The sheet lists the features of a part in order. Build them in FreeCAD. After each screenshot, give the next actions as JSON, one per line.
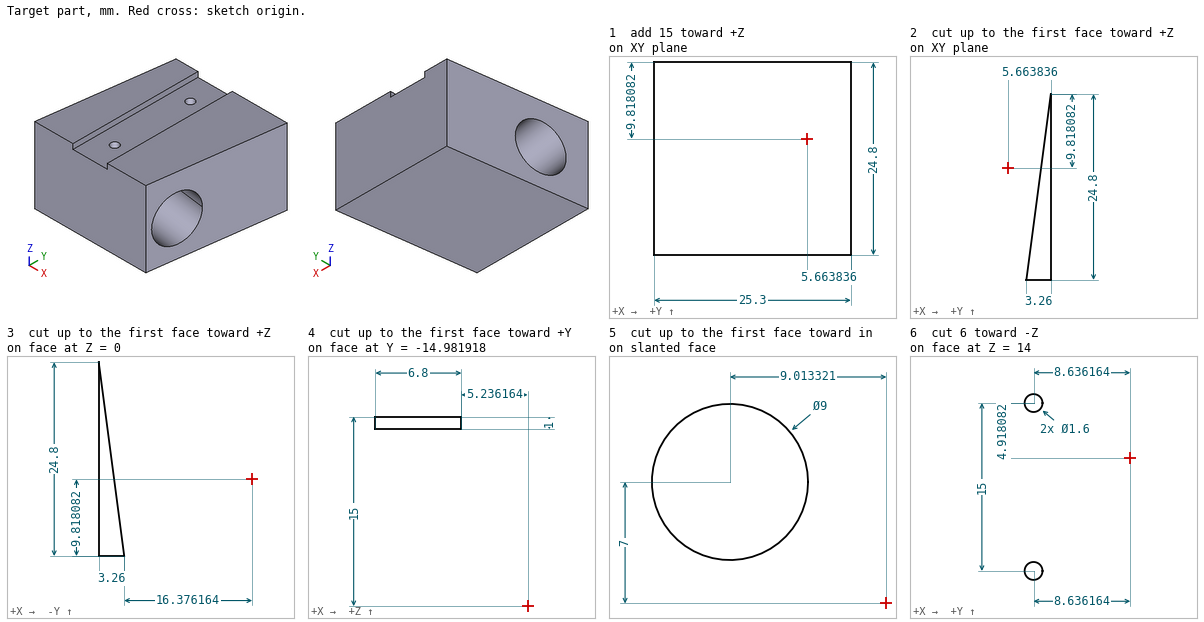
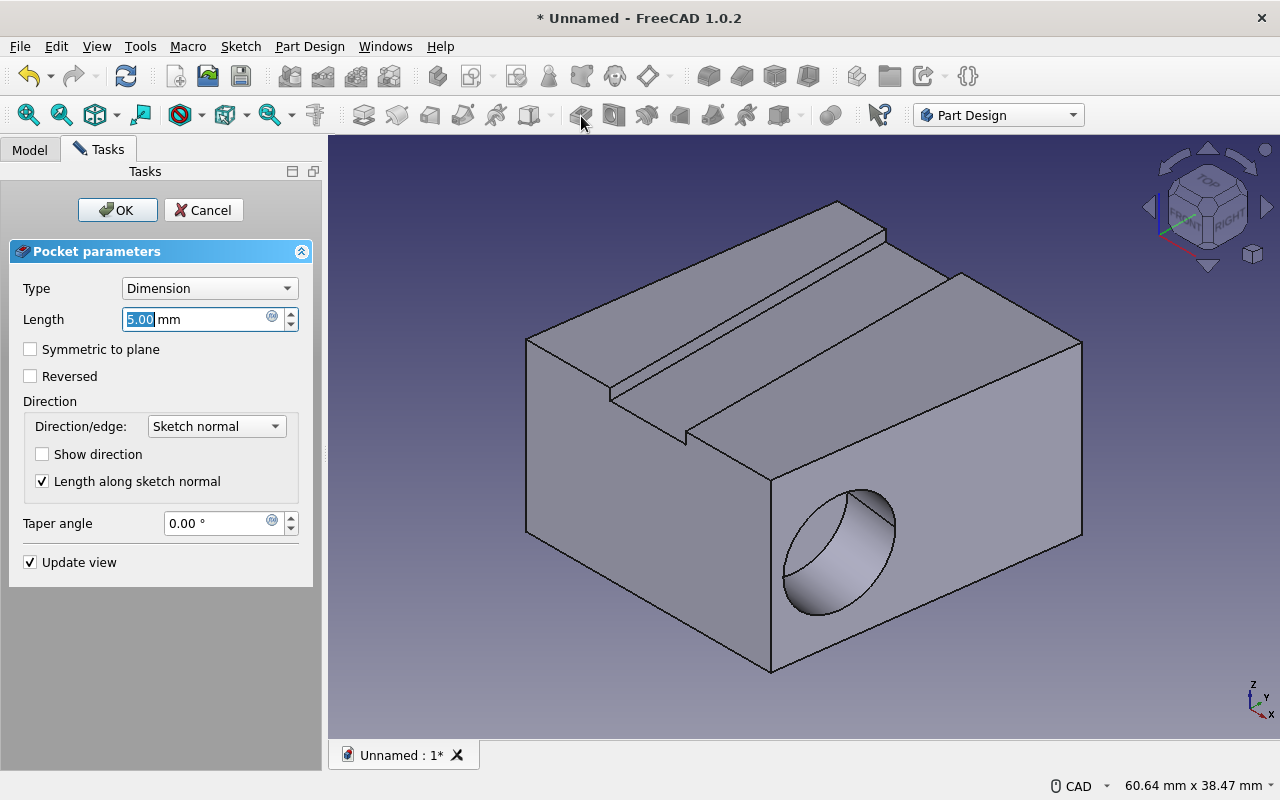
{"action": "left_click", "coordinate": [210, 288]}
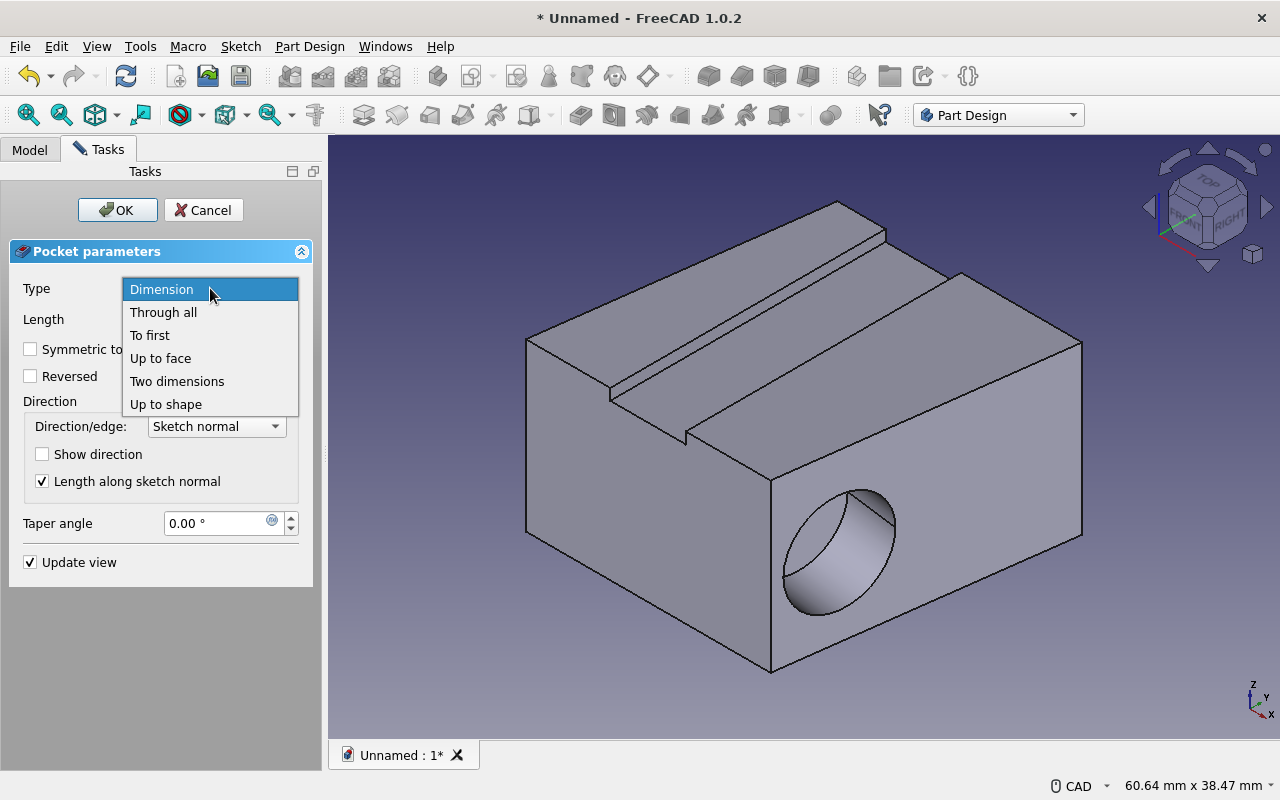
{"action": "left_click", "coordinate": [208, 336]}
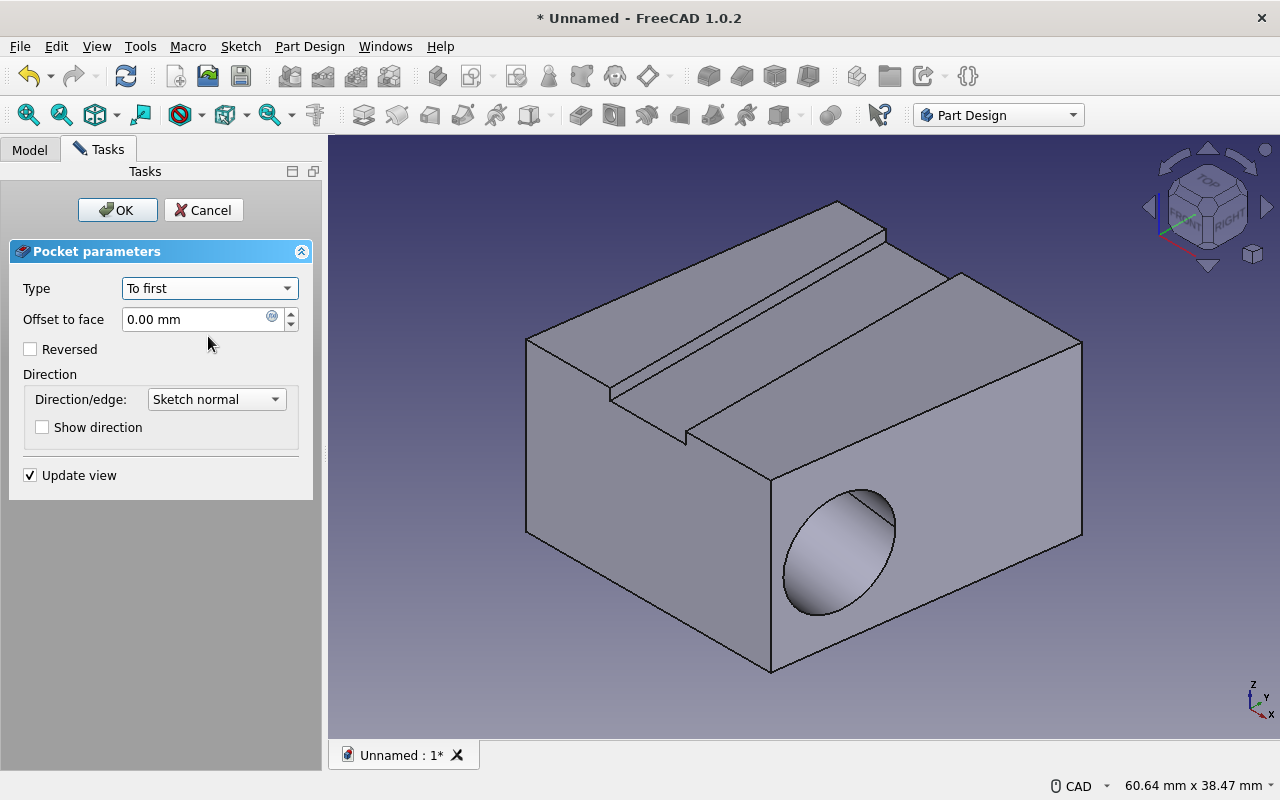
{"action": "left_click", "coordinate": [118, 210]}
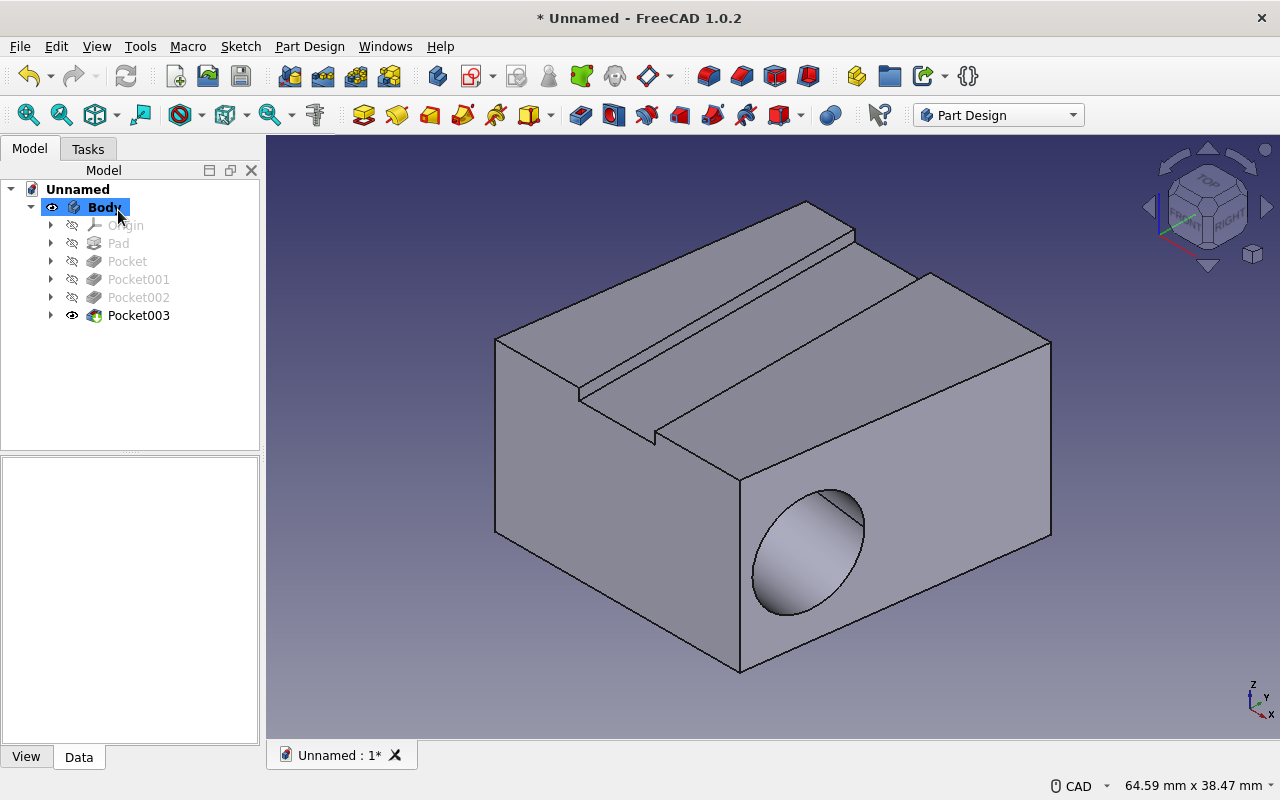
{"action": "left_click", "coordinate": [833, 297]}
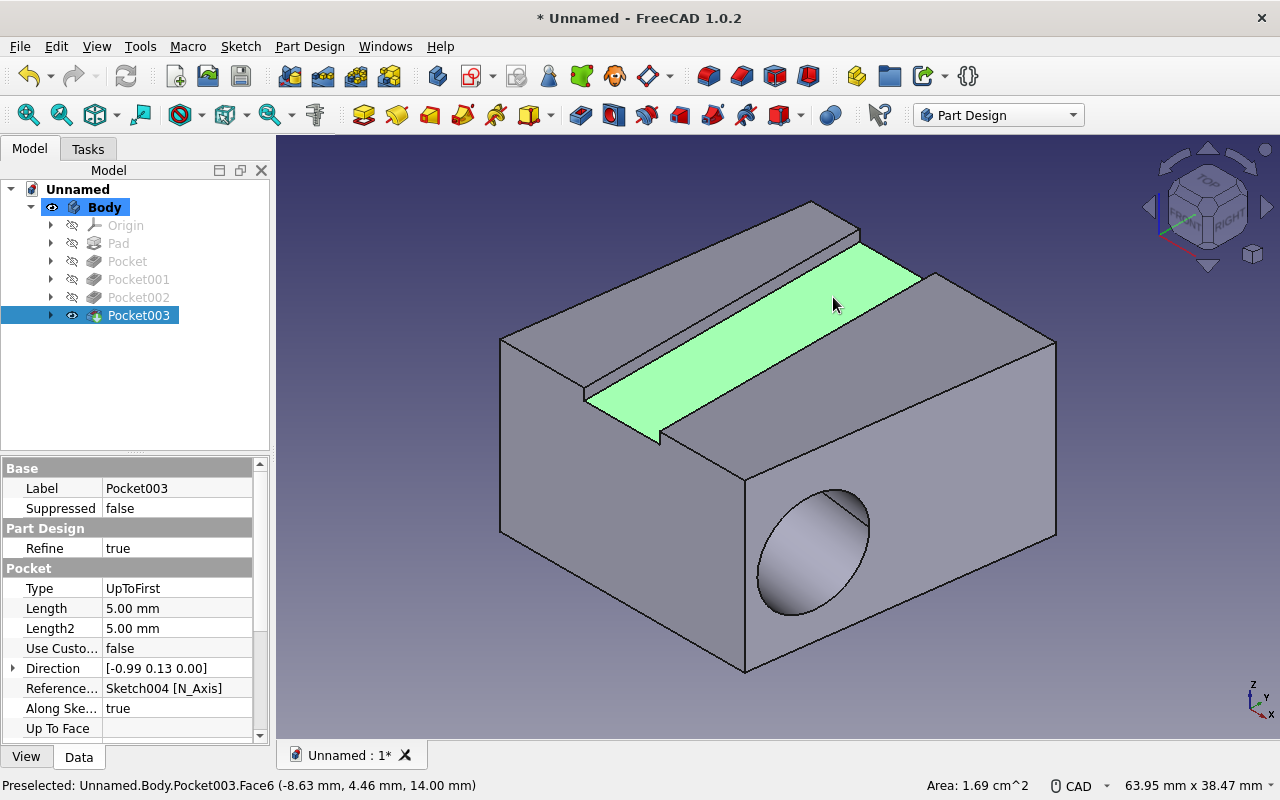
{"action": "left_click", "coordinate": [470, 76]}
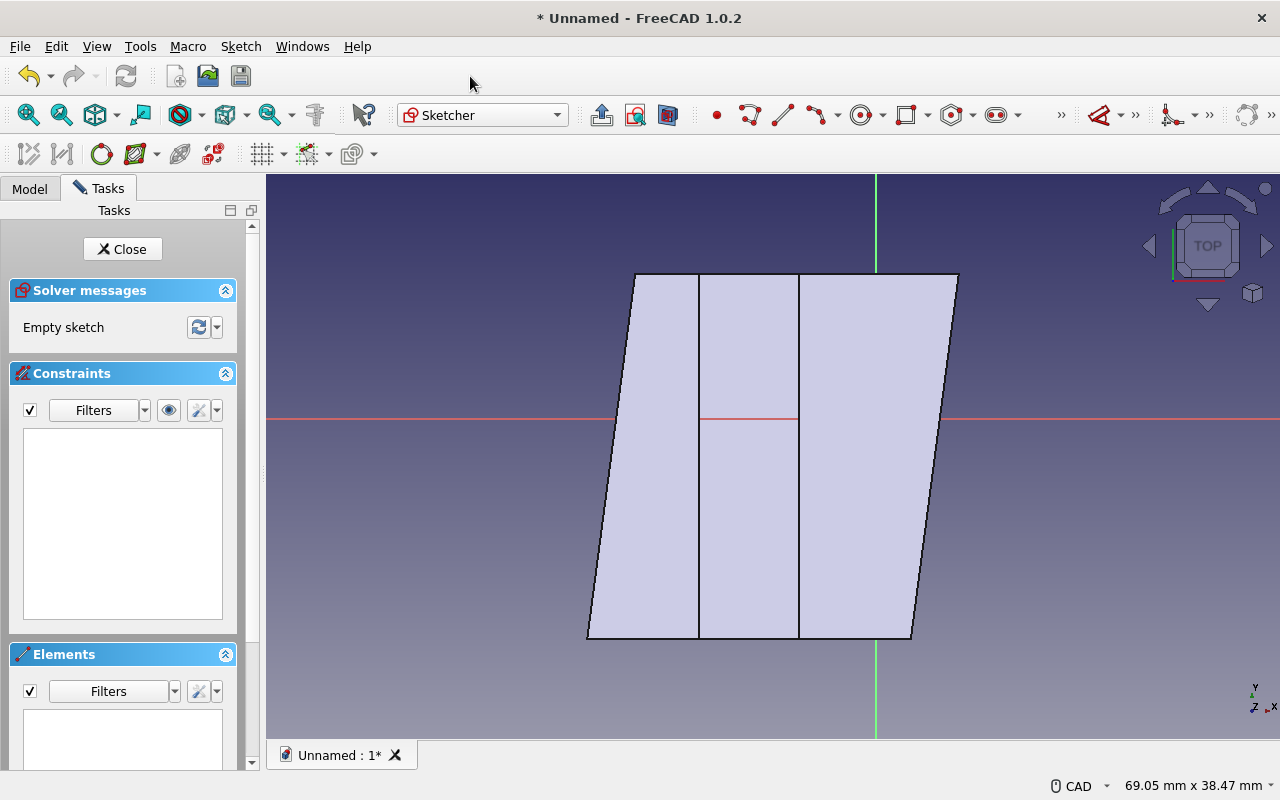
{"action": "left_click", "coordinate": [668, 116]}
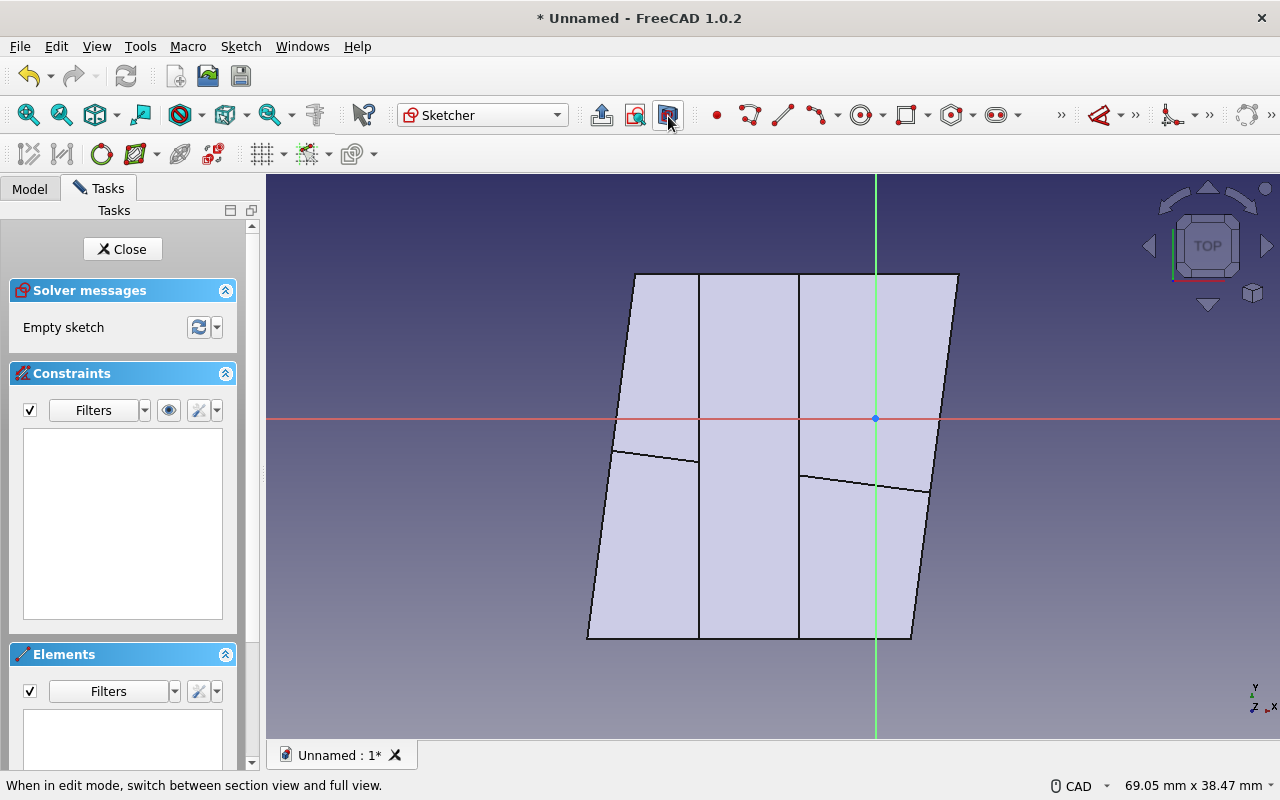
{"action": "scroll", "coordinate": [1013, 456], "scroll_direction": "up", "scroll_amount": 2}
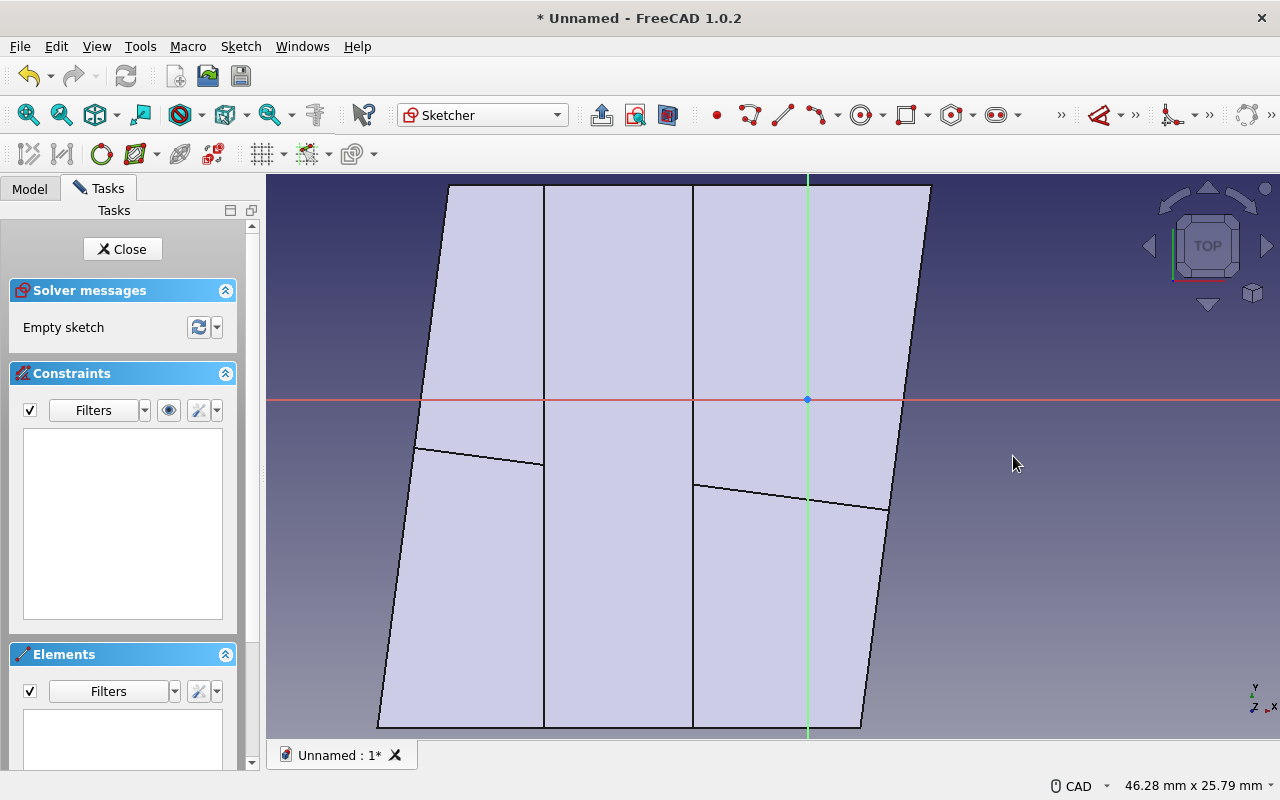
{"action": "left_click", "coordinate": [860, 116]}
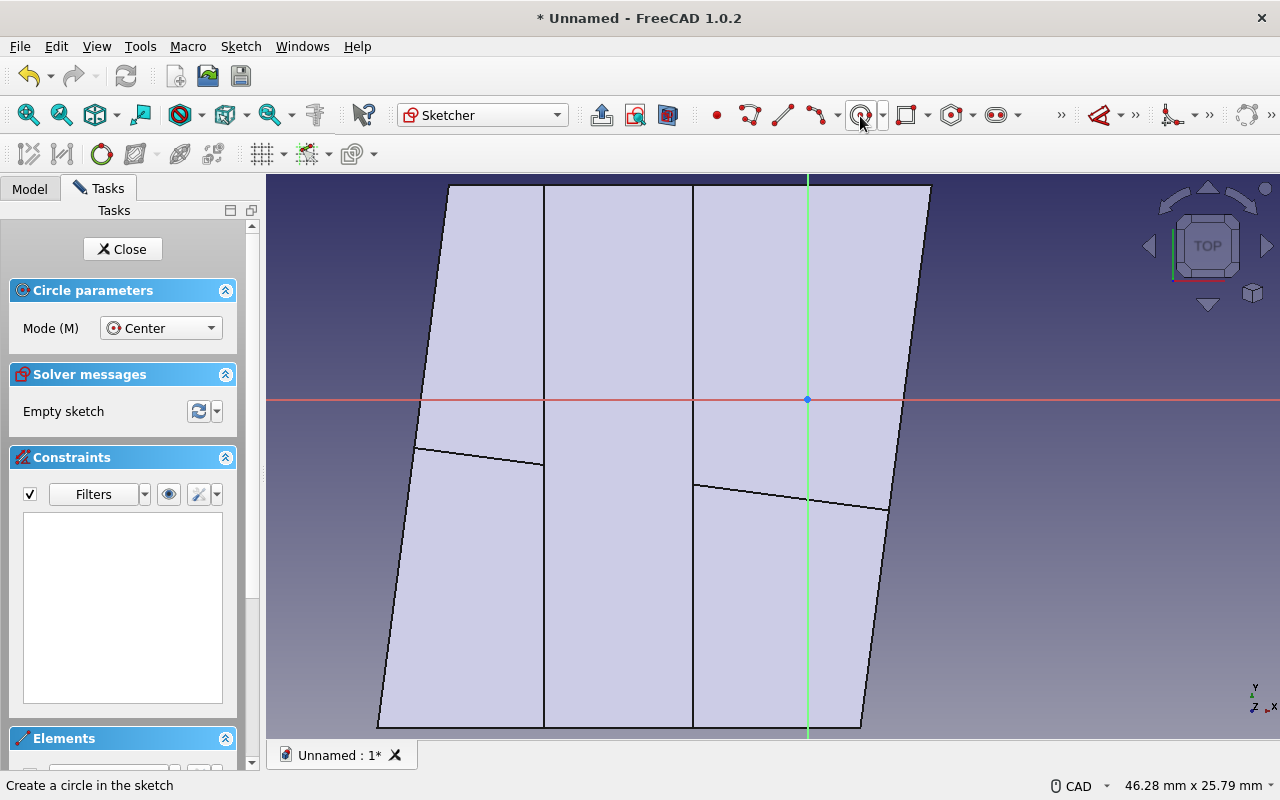
{"action": "scroll", "coordinate": [618, 292], "scroll_direction": "up", "scroll_amount": 2}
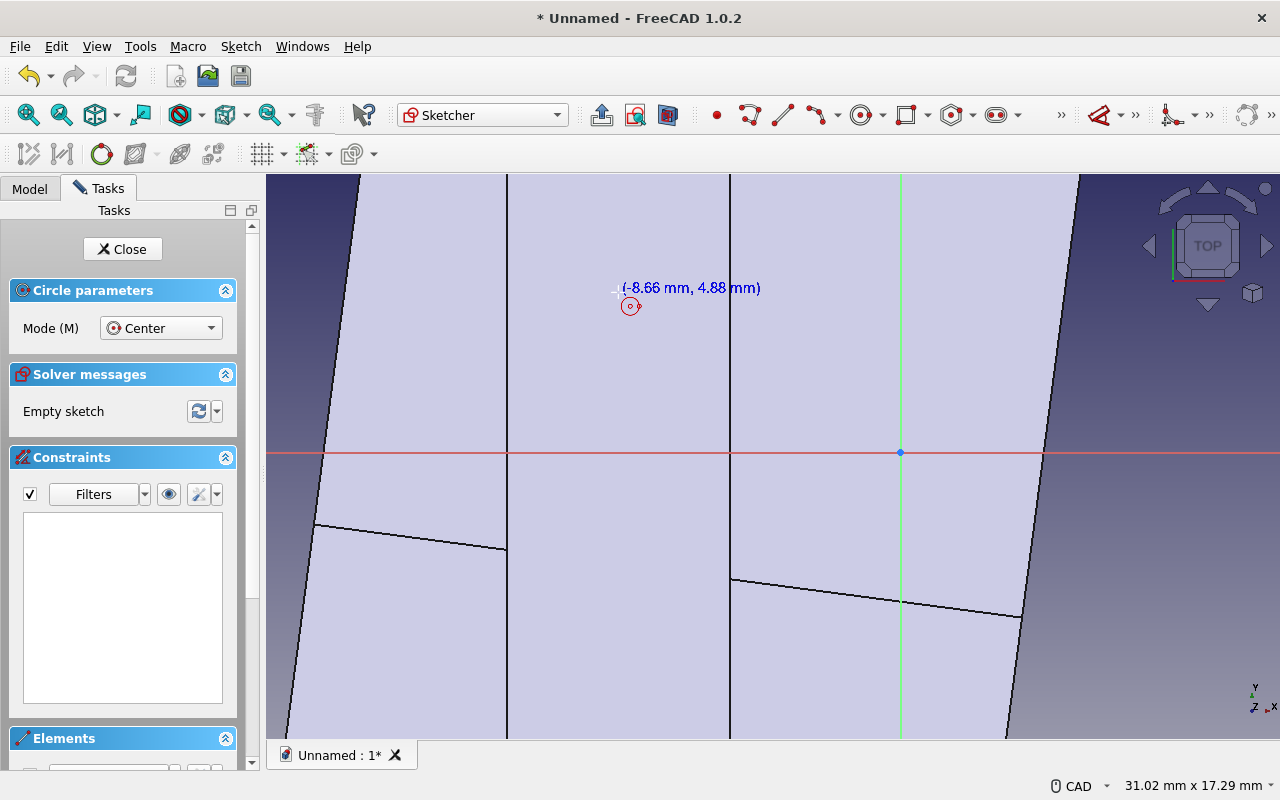
{"action": "left_click", "coordinate": [619, 292]}
{"action": "mouse_move", "coordinate": [637, 274]}